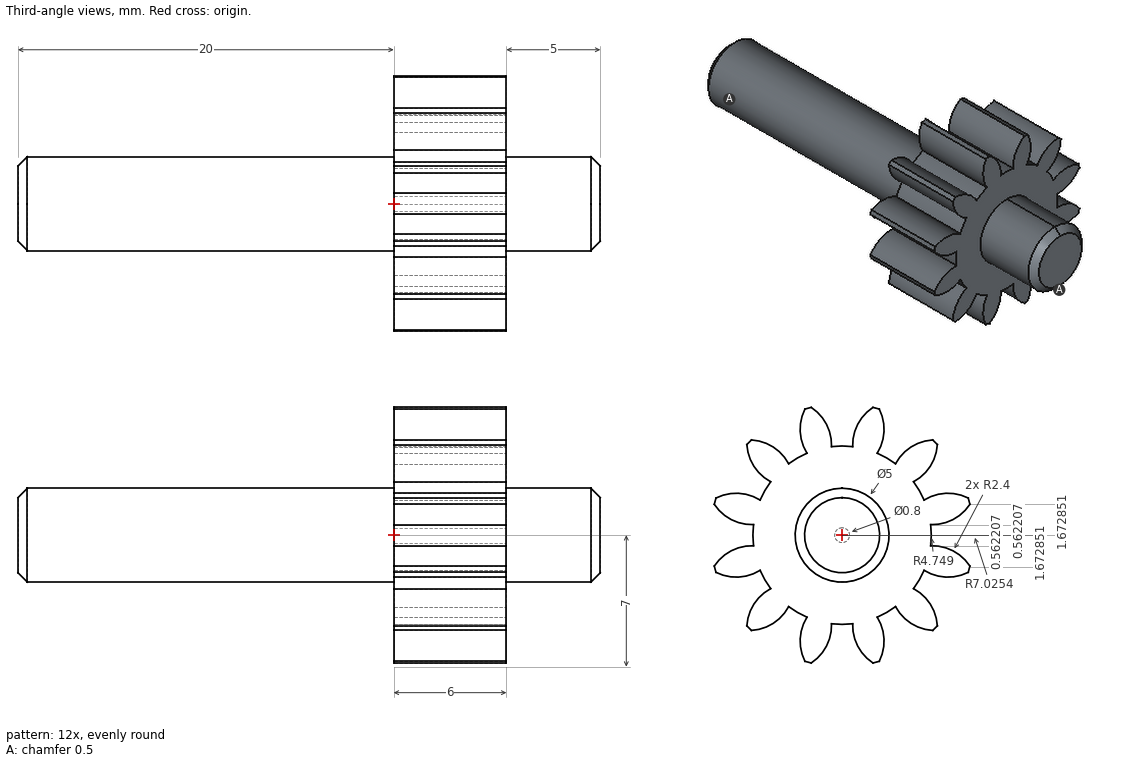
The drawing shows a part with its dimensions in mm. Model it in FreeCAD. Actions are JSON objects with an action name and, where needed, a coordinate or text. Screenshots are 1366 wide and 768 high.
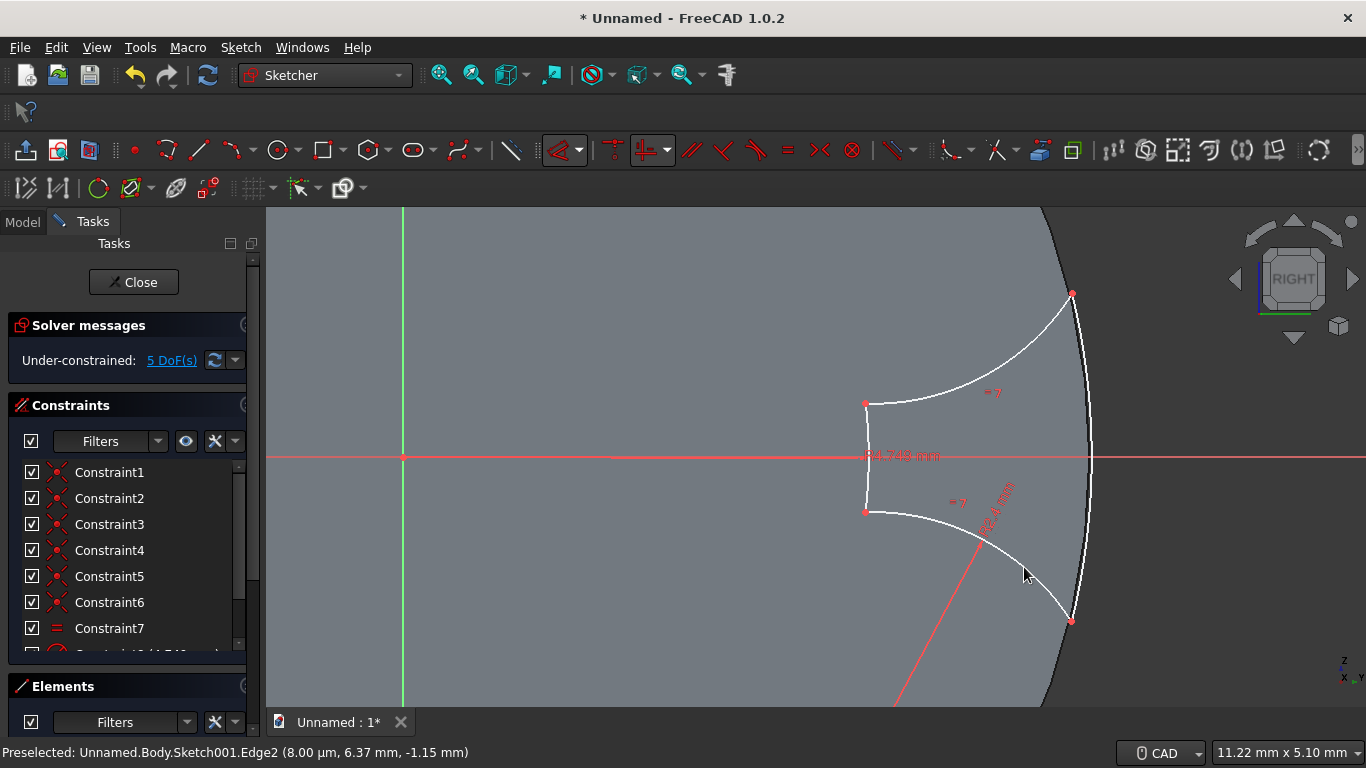
{"action": "left_click", "coordinate": [1088, 524]}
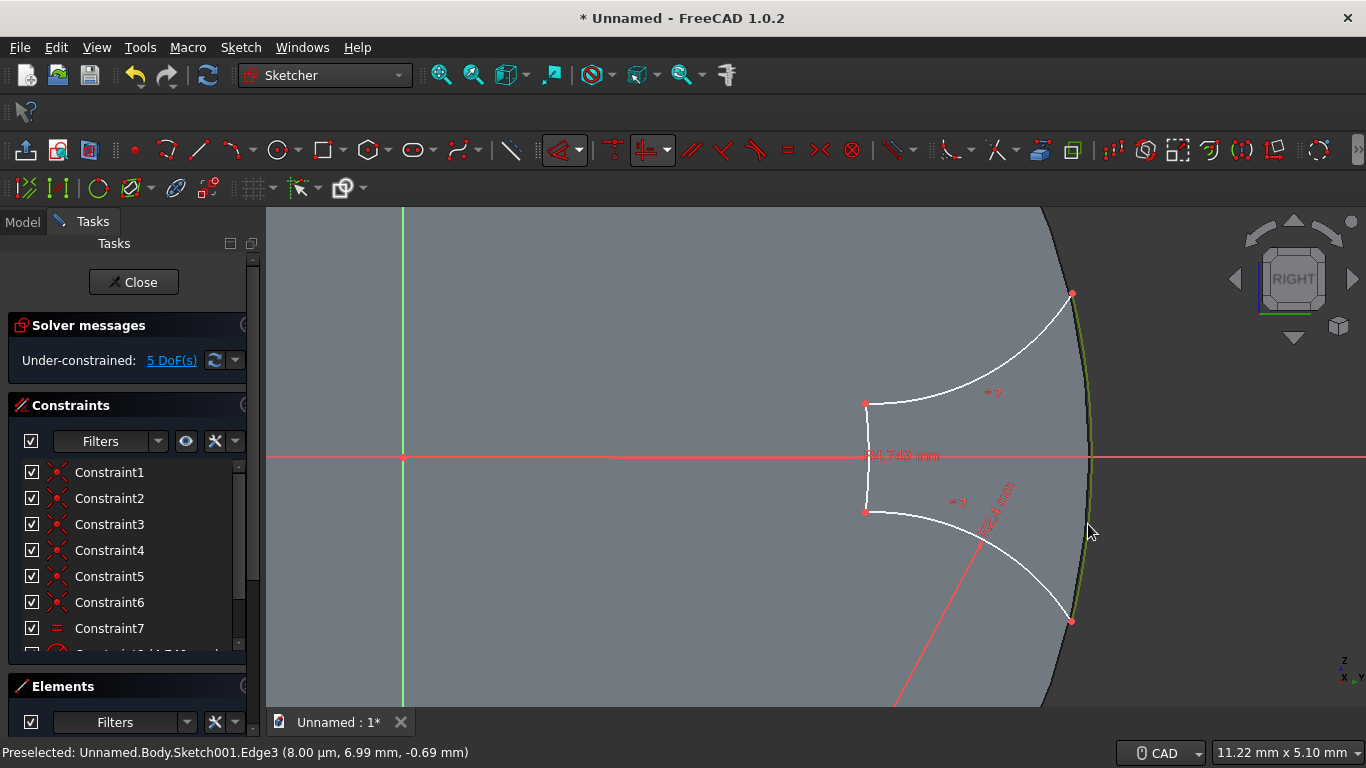
{"action": "key", "text": "k r"}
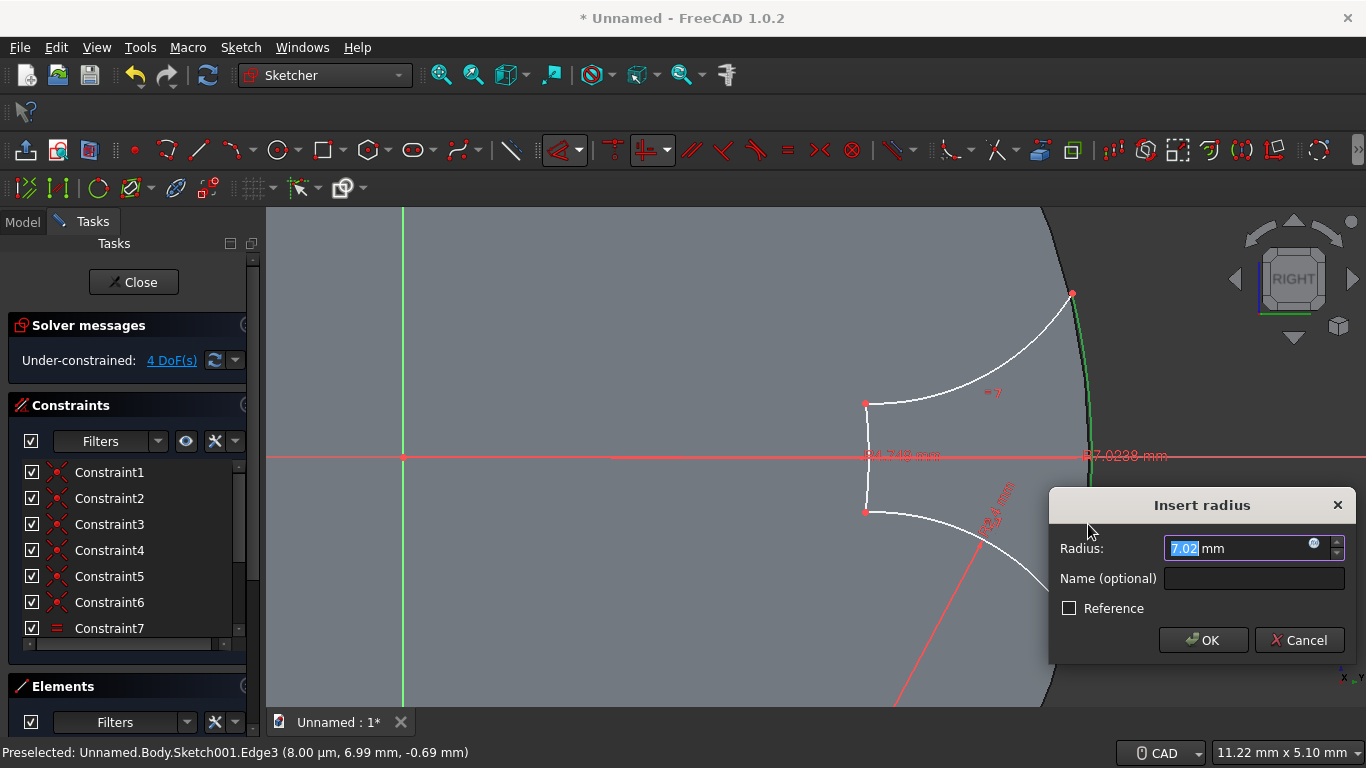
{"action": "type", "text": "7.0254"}
{"action": "key", "text": "Return"}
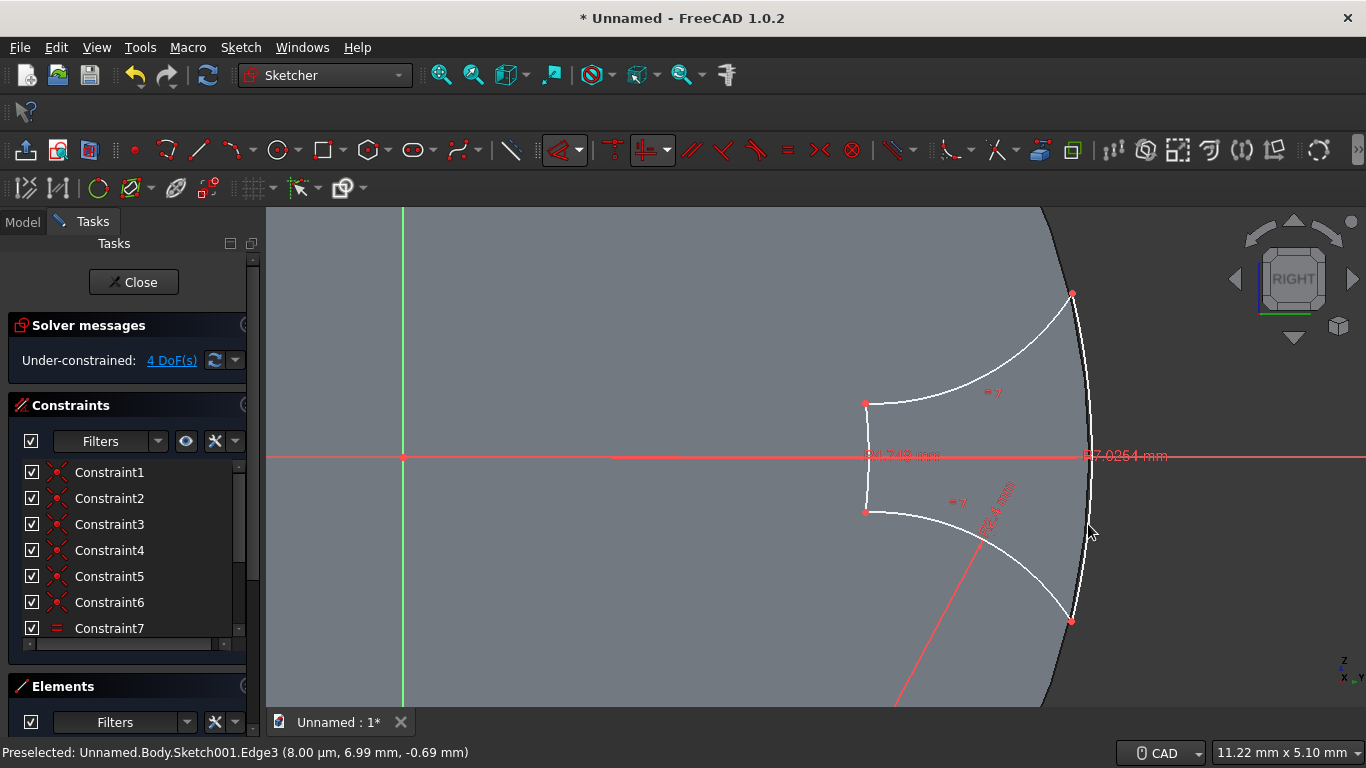
{"action": "left_click", "coordinate": [865, 512]}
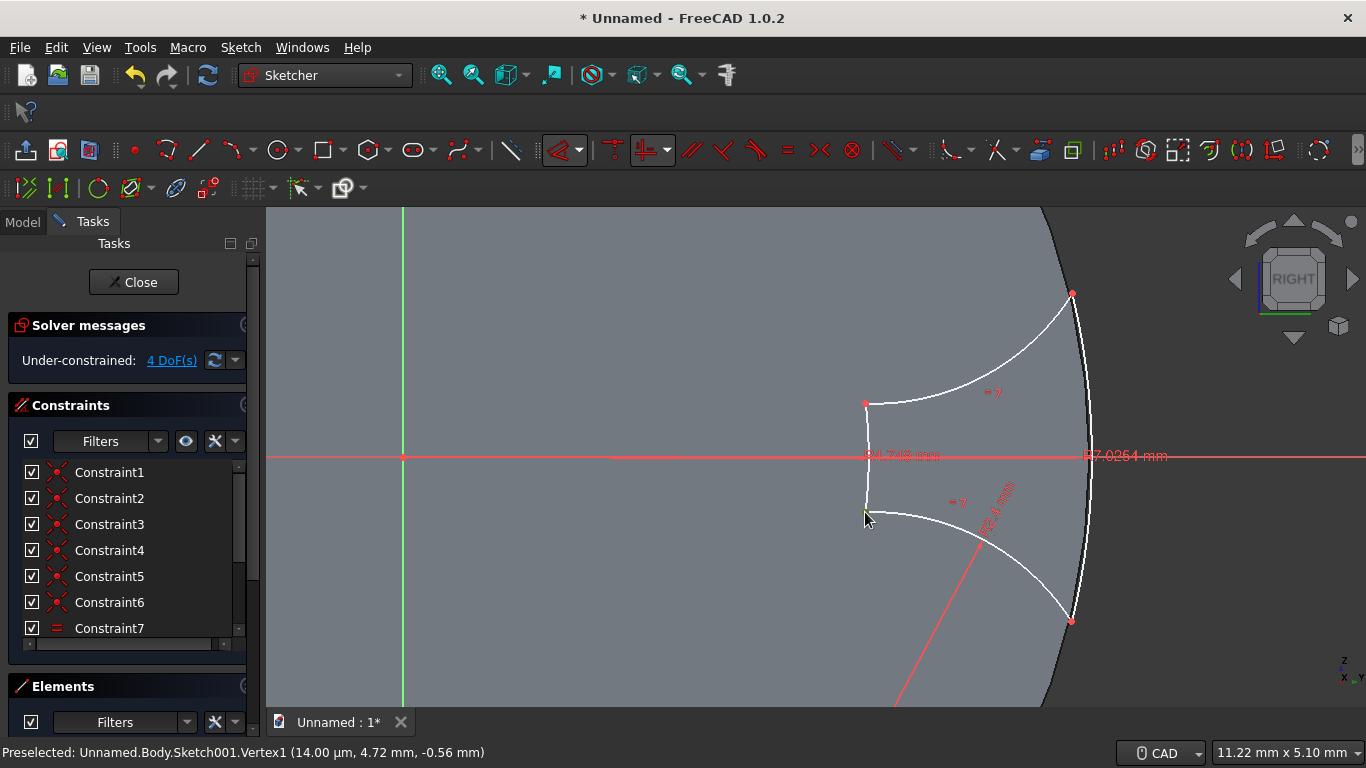
{"action": "key", "text": "i"}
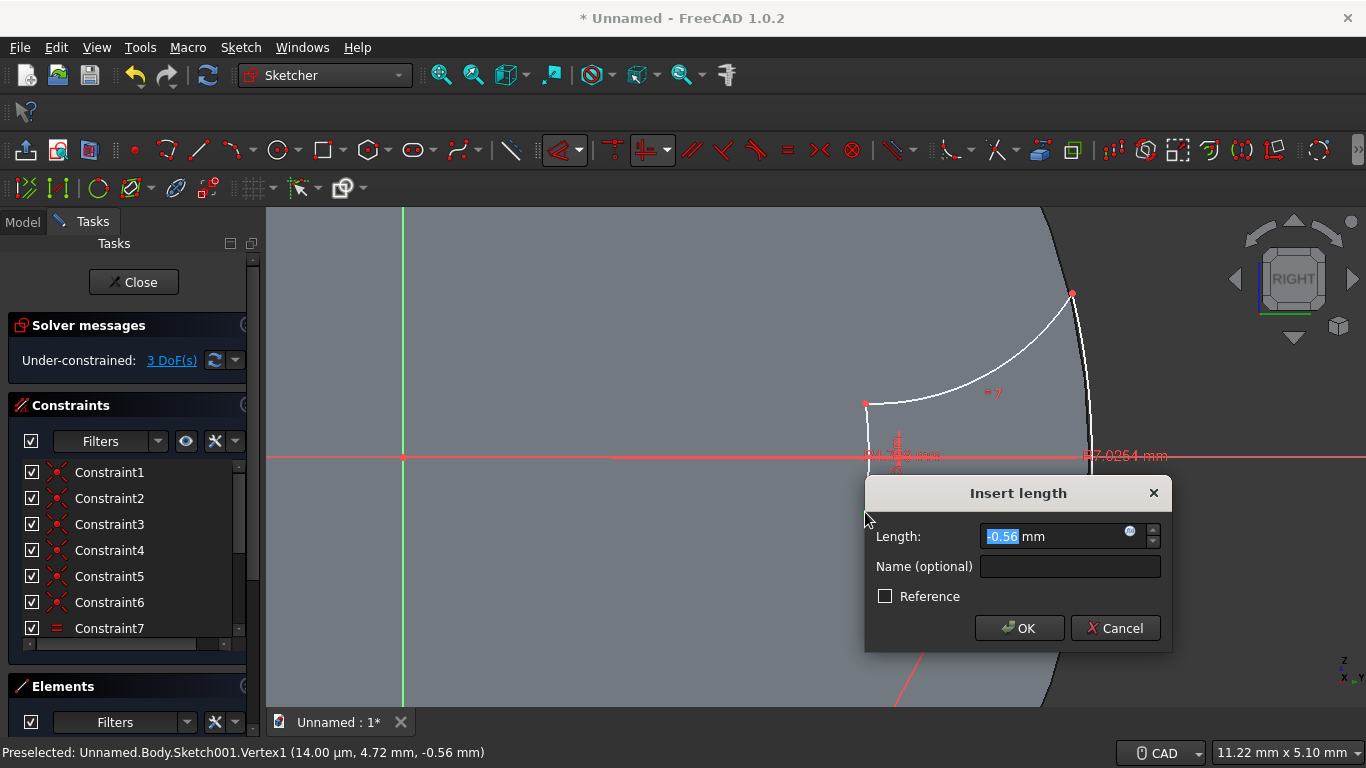
{"action": "type", "text": "-0.562207"}
{"action": "key", "text": "Return"}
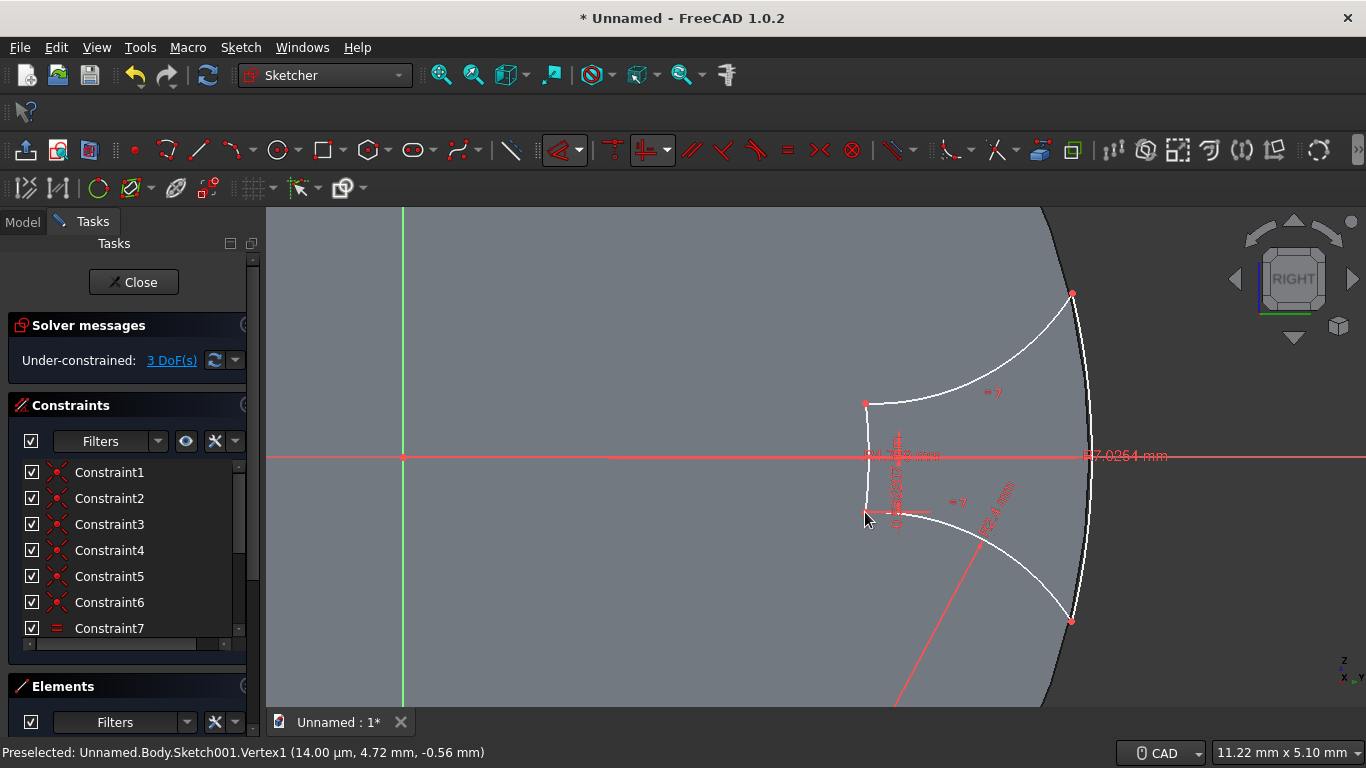
{"action": "left_click", "coordinate": [866, 404]}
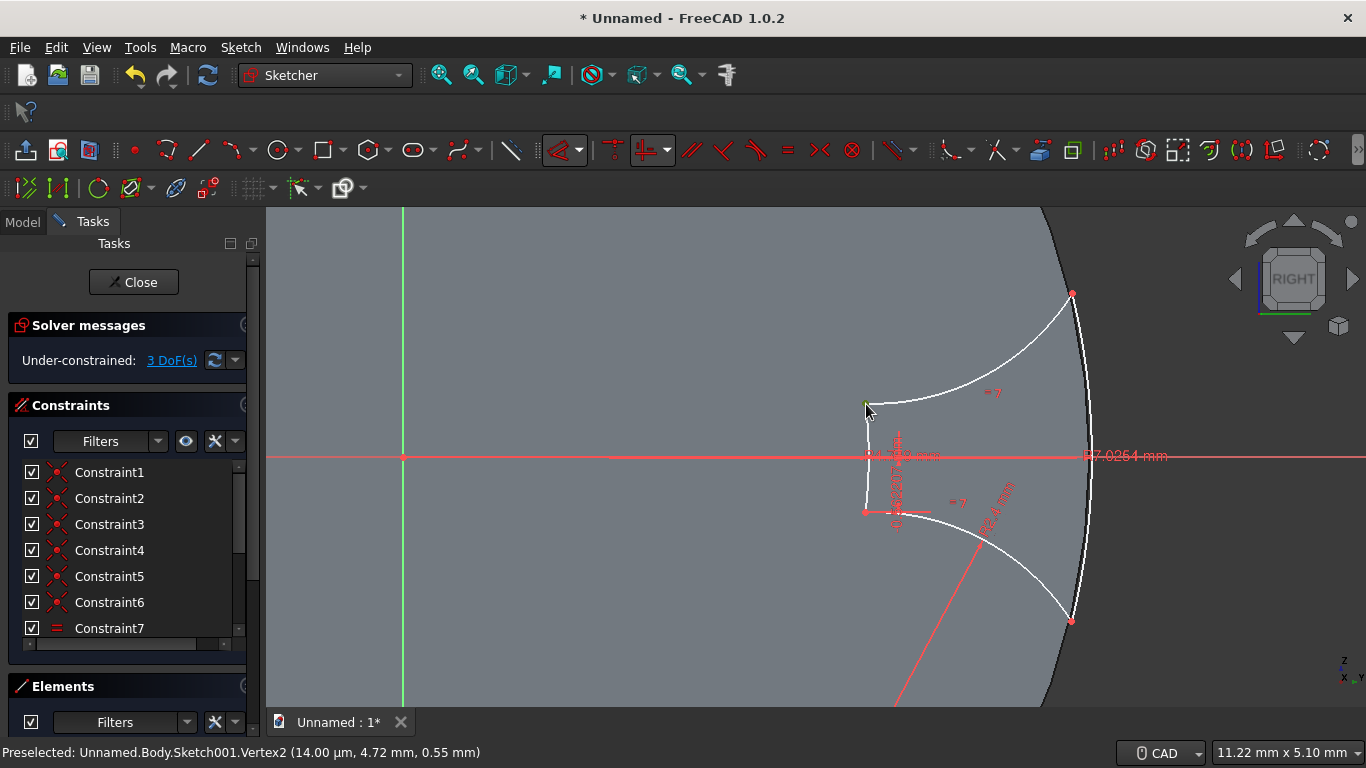
{"action": "key", "text": "i"}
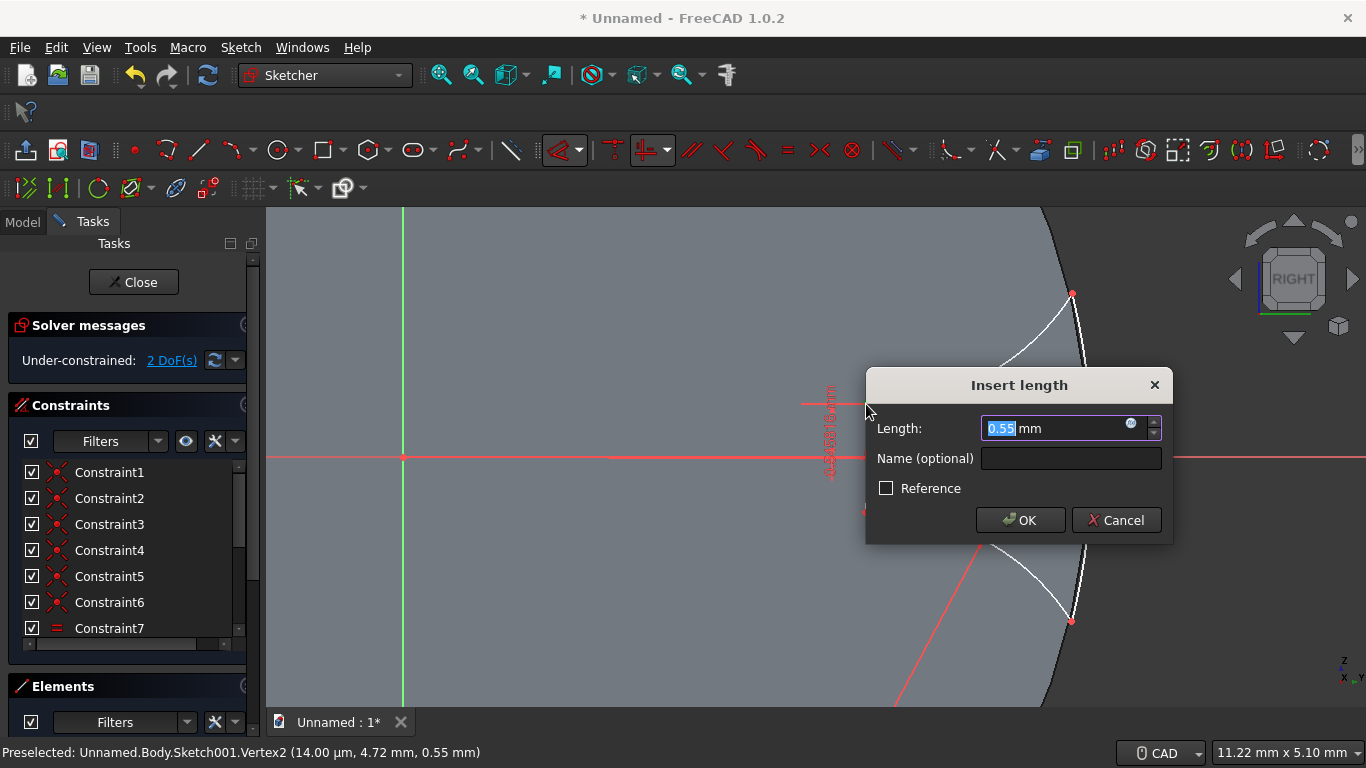
{"action": "type", "text": "0.562207"}
{"action": "key", "text": "Return"}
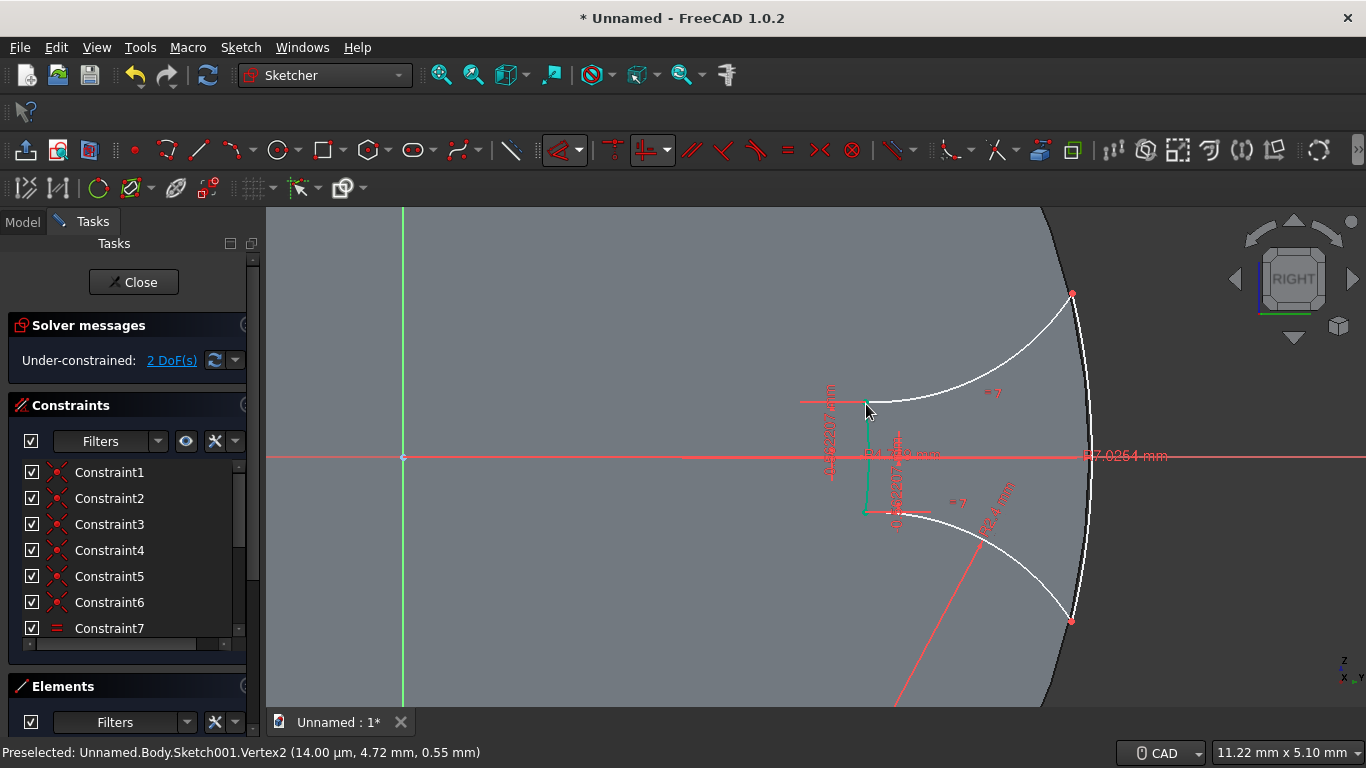
{"action": "left_click", "coordinate": [1072, 622]}